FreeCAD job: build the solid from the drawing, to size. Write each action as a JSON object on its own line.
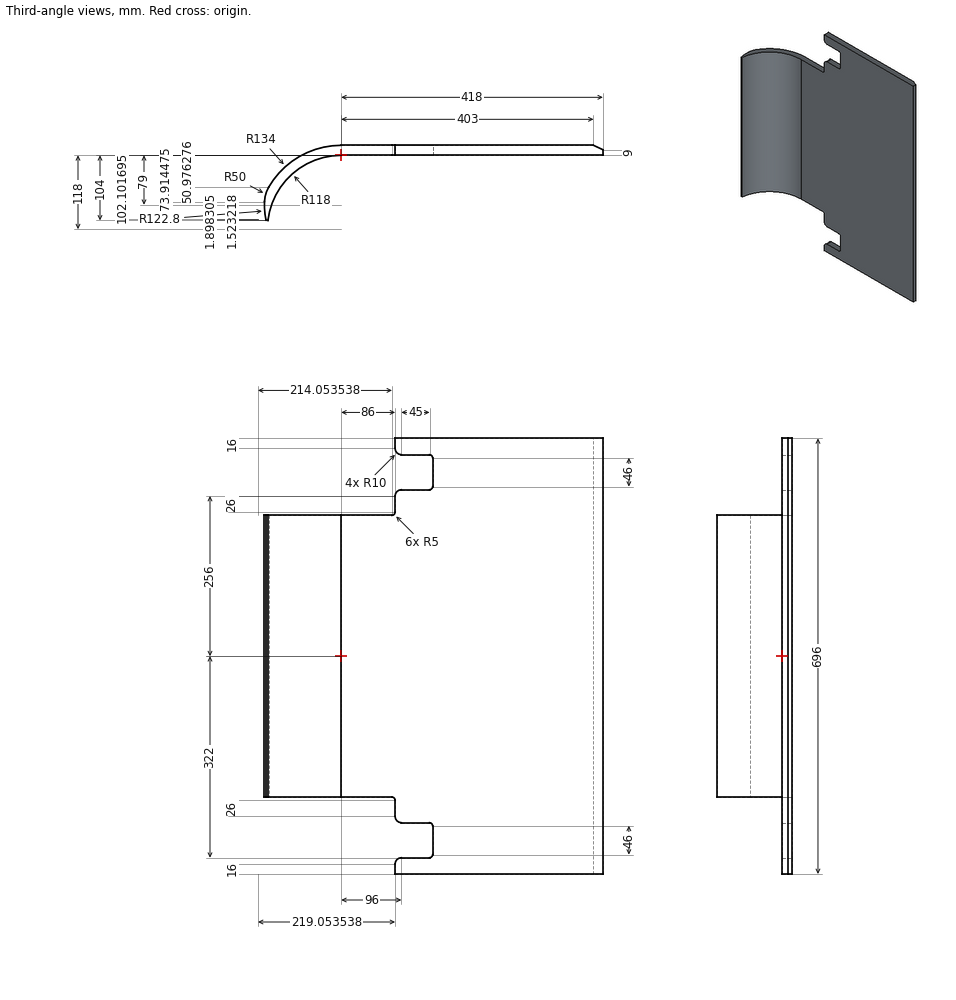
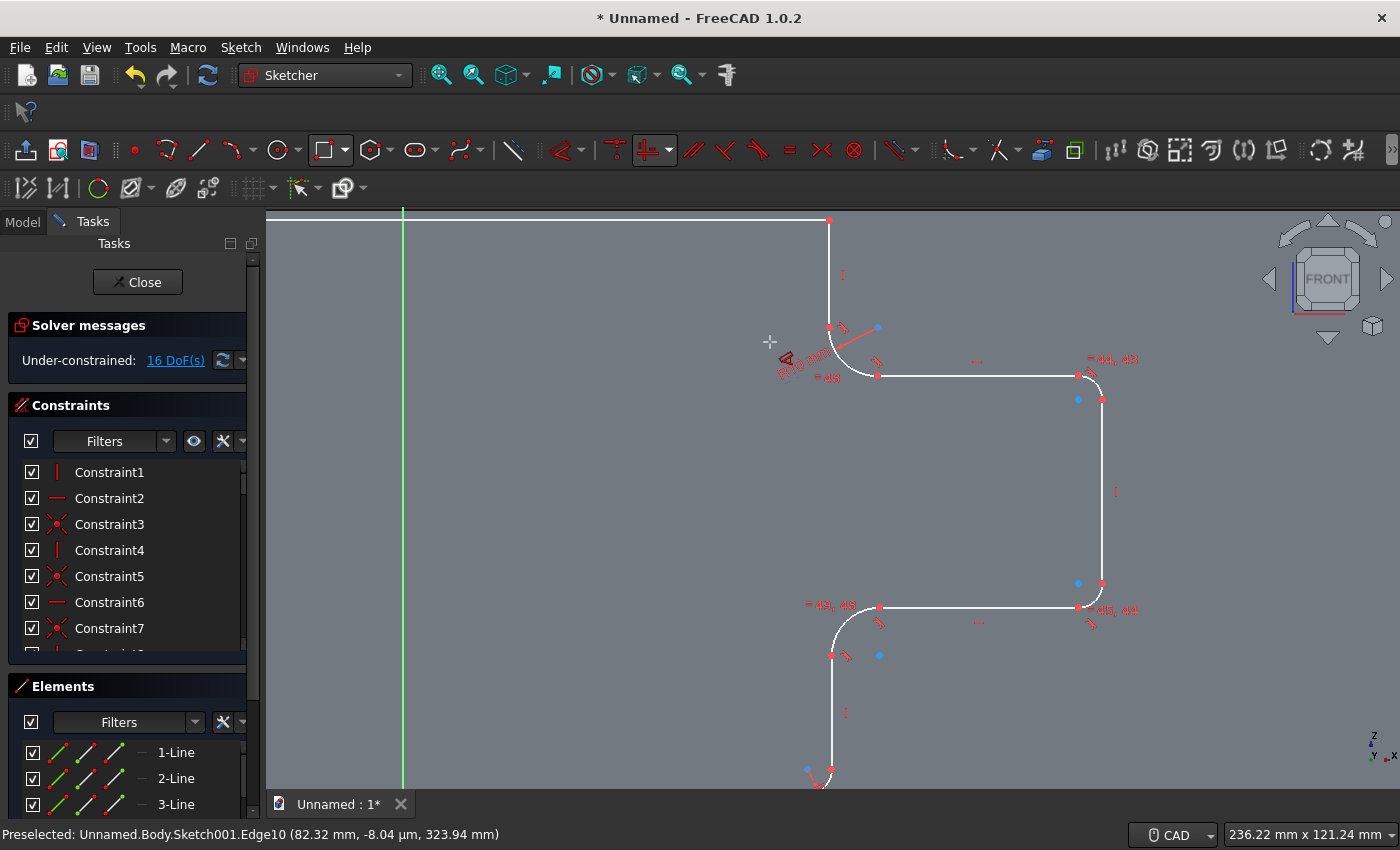
{"action": "left_click", "coordinate": [832, 690]}
{"action": "left_click", "coordinate": [866, 708]}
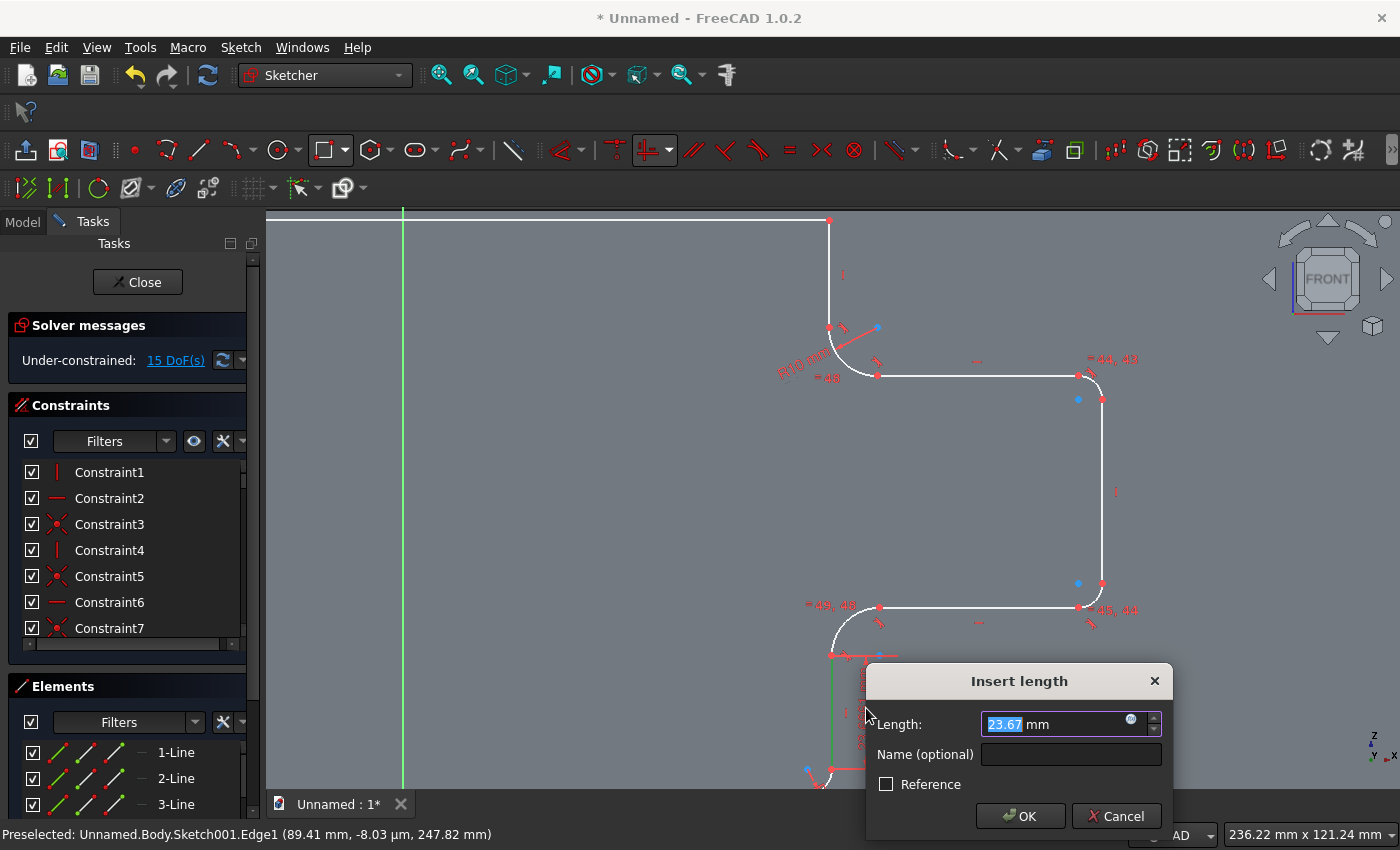
{"action": "type", "text": "26"}
{"action": "key", "text": "Return"}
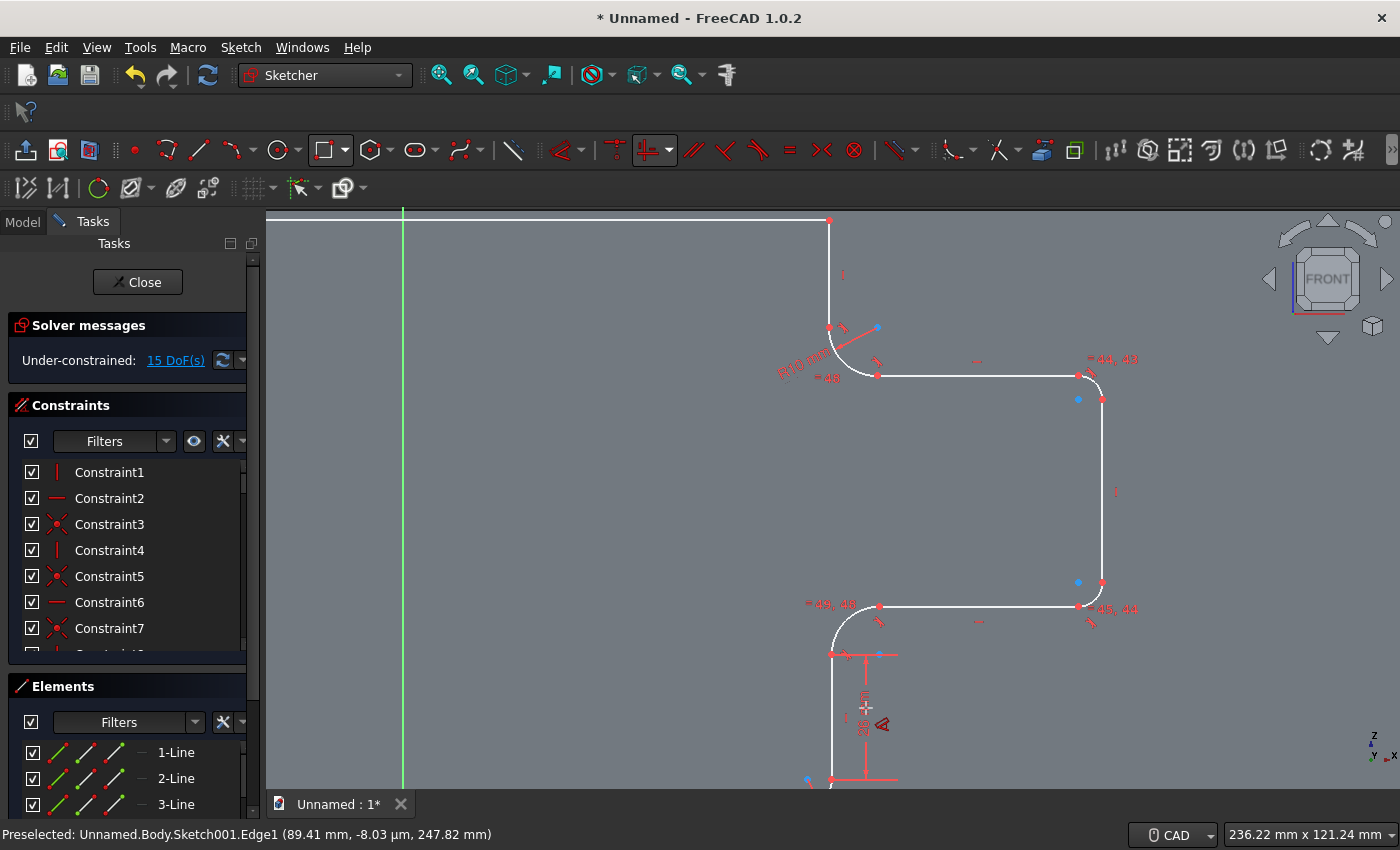
{"action": "left_click", "coordinate": [829, 253]}
{"action": "left_click", "coordinate": [863, 281]}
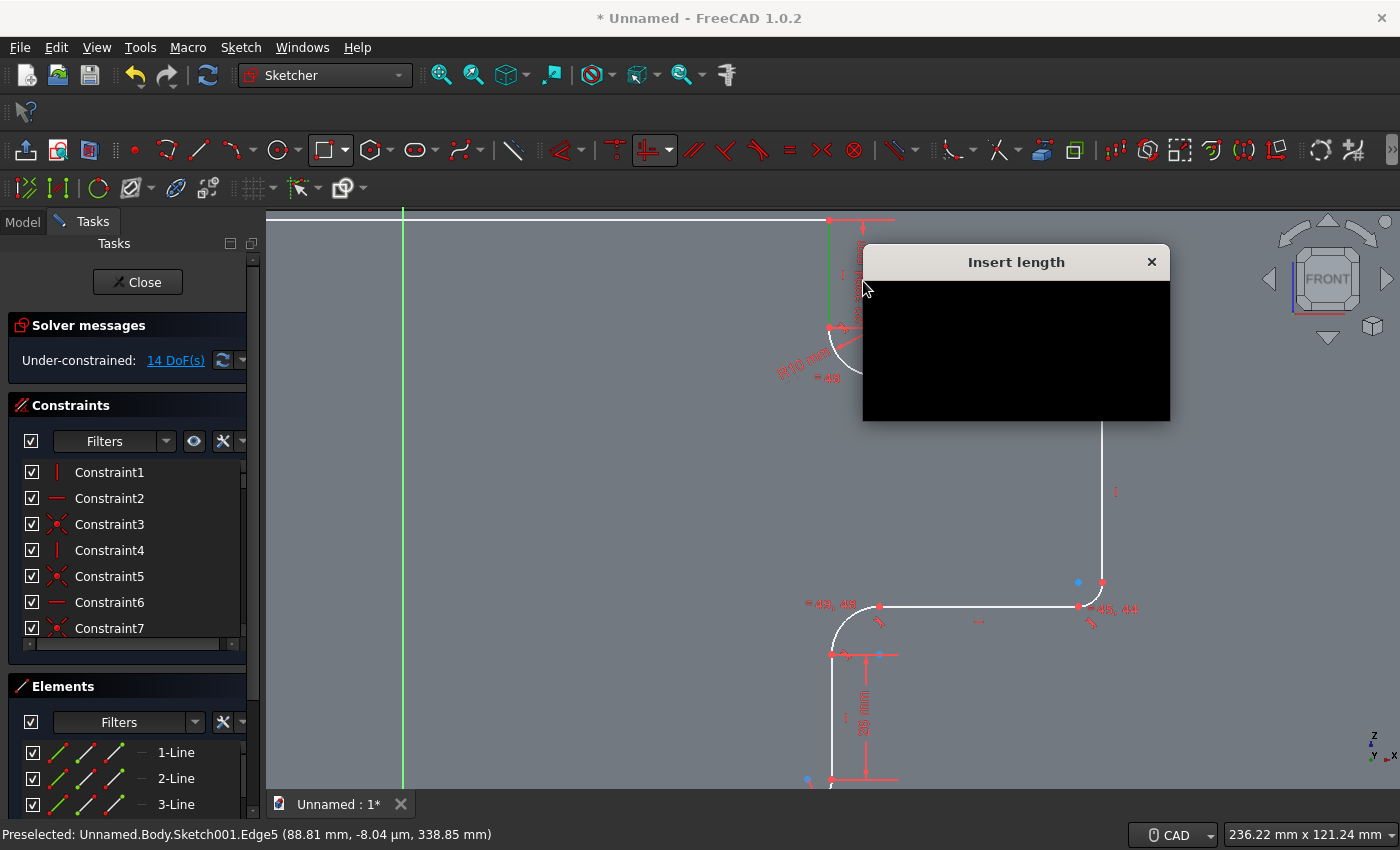
{"action": "type", "text": "16"}
{"action": "key", "text": "Return"}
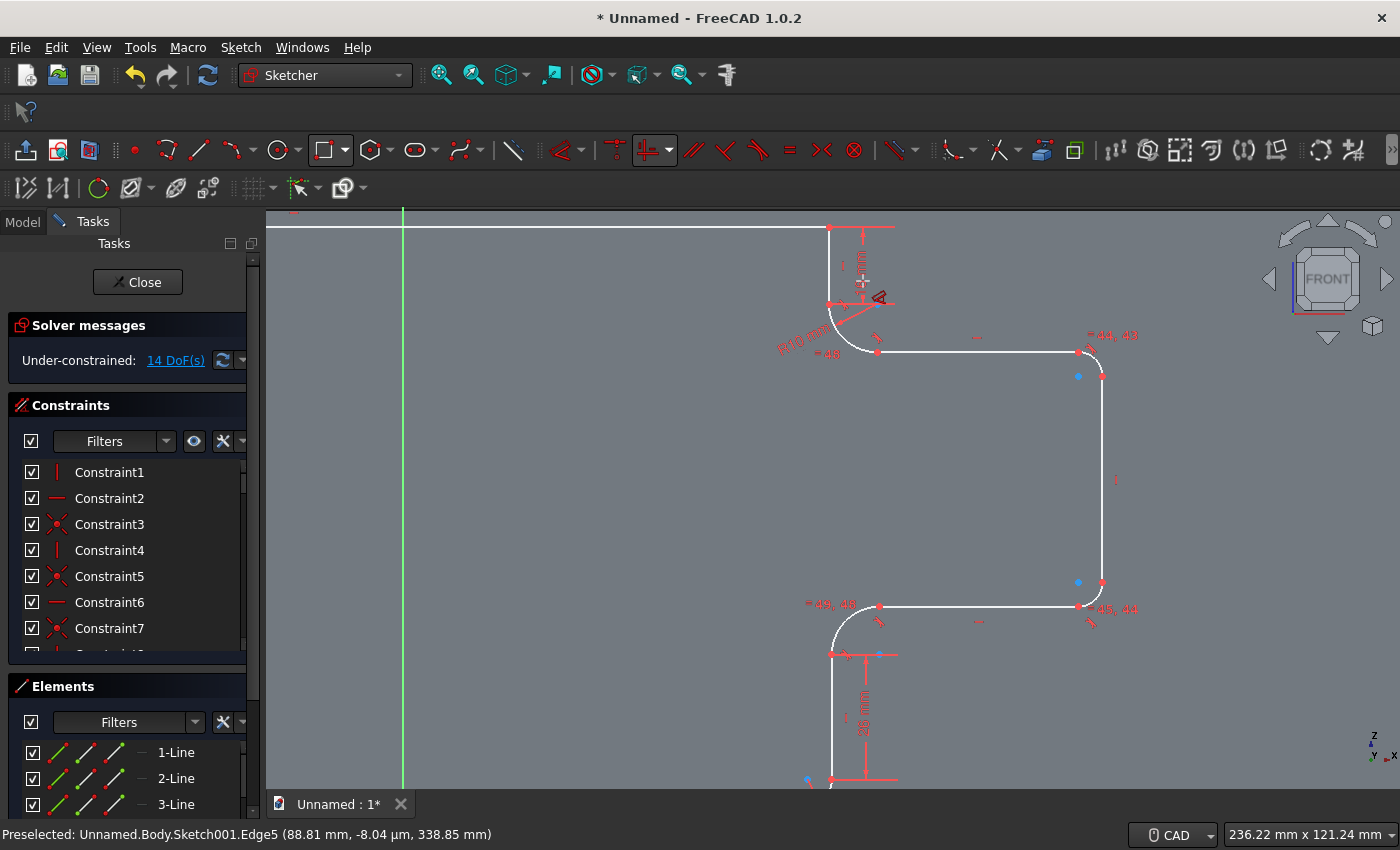
{"action": "scroll", "coordinate": [806, 326], "scroll_direction": "down", "scroll_amount": 11}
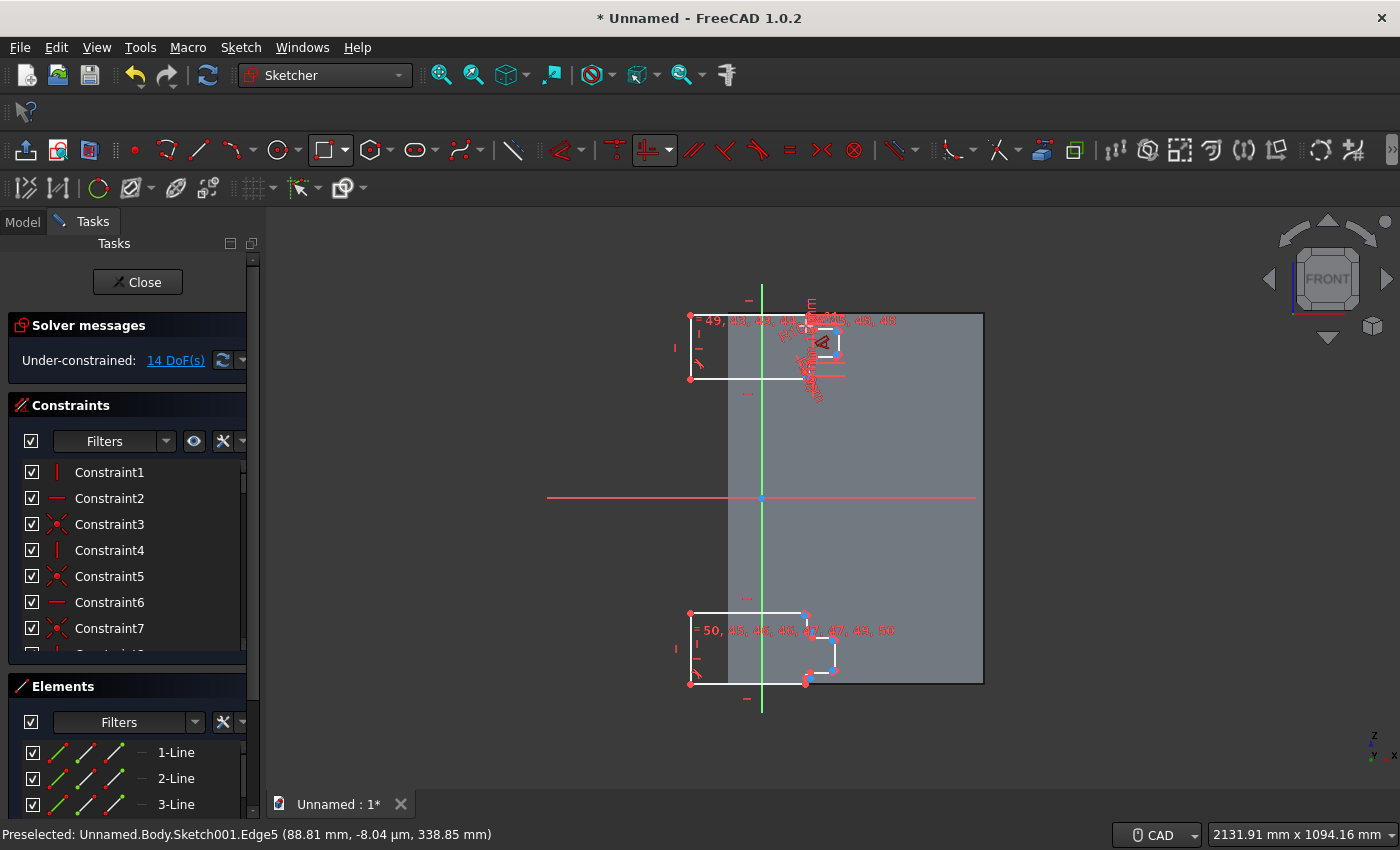
{"action": "scroll", "coordinate": [821, 329], "scroll_direction": "up", "scroll_amount": 4}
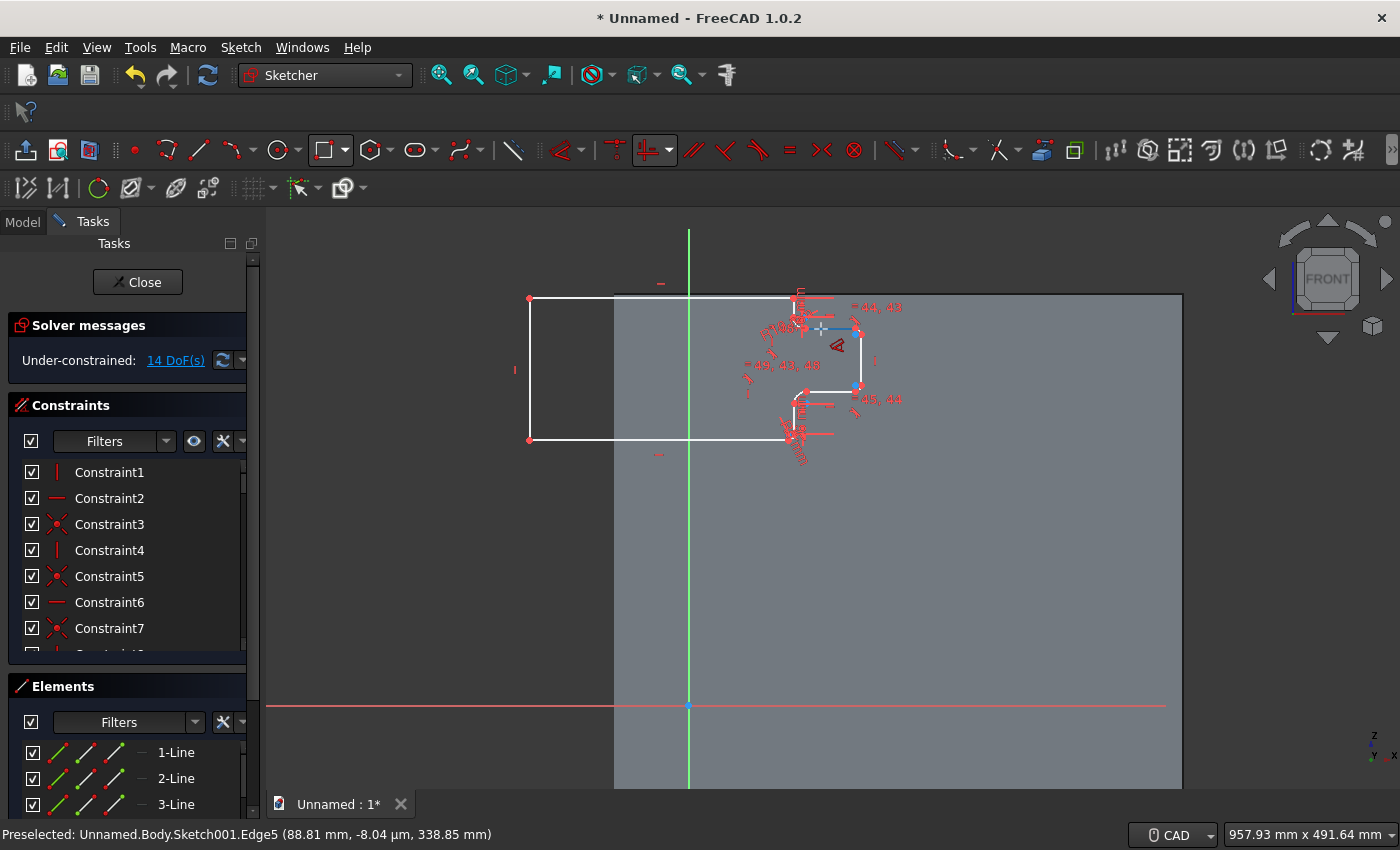
{"action": "left_click", "coordinate": [820, 329]}
{"action": "left_click", "coordinate": [830, 363]}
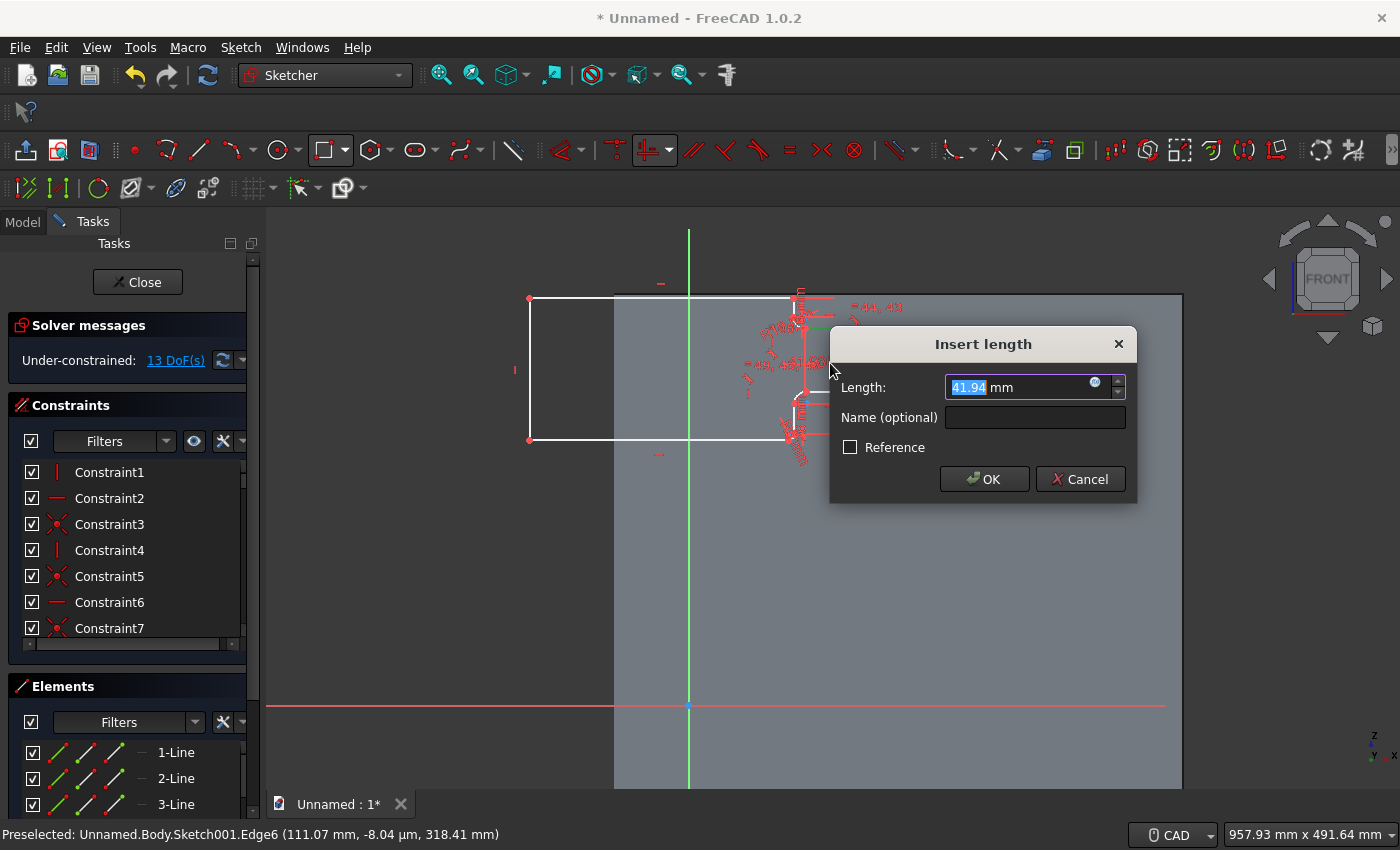
{"action": "type", "text": "45"}
{"action": "key", "text": "Return"}